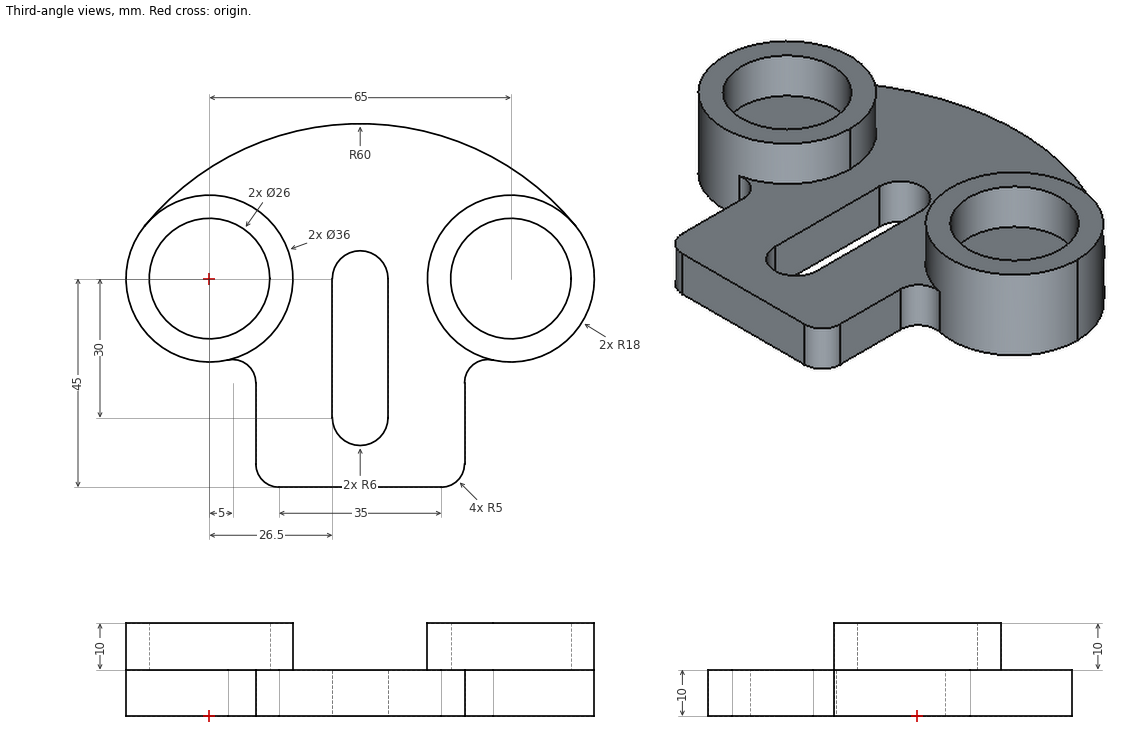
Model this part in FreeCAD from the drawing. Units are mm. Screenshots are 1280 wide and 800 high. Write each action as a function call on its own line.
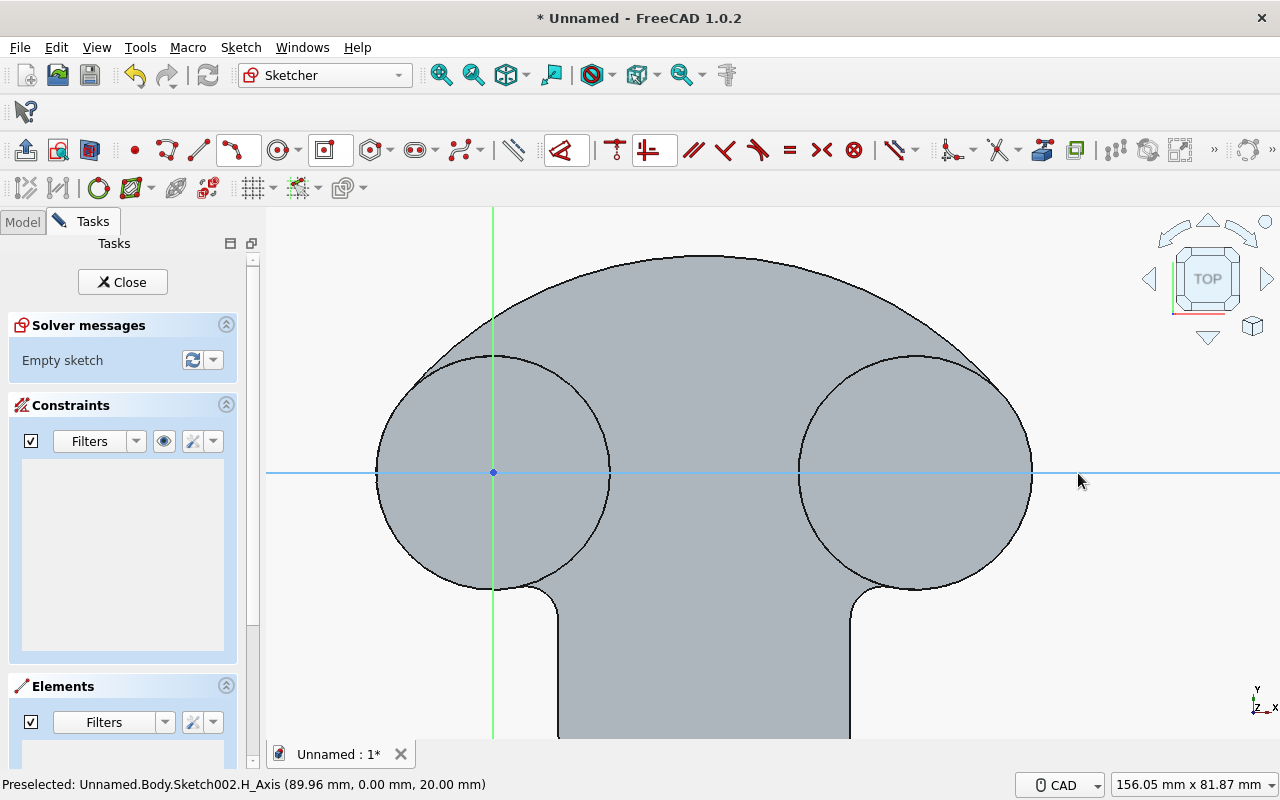
click(278, 150)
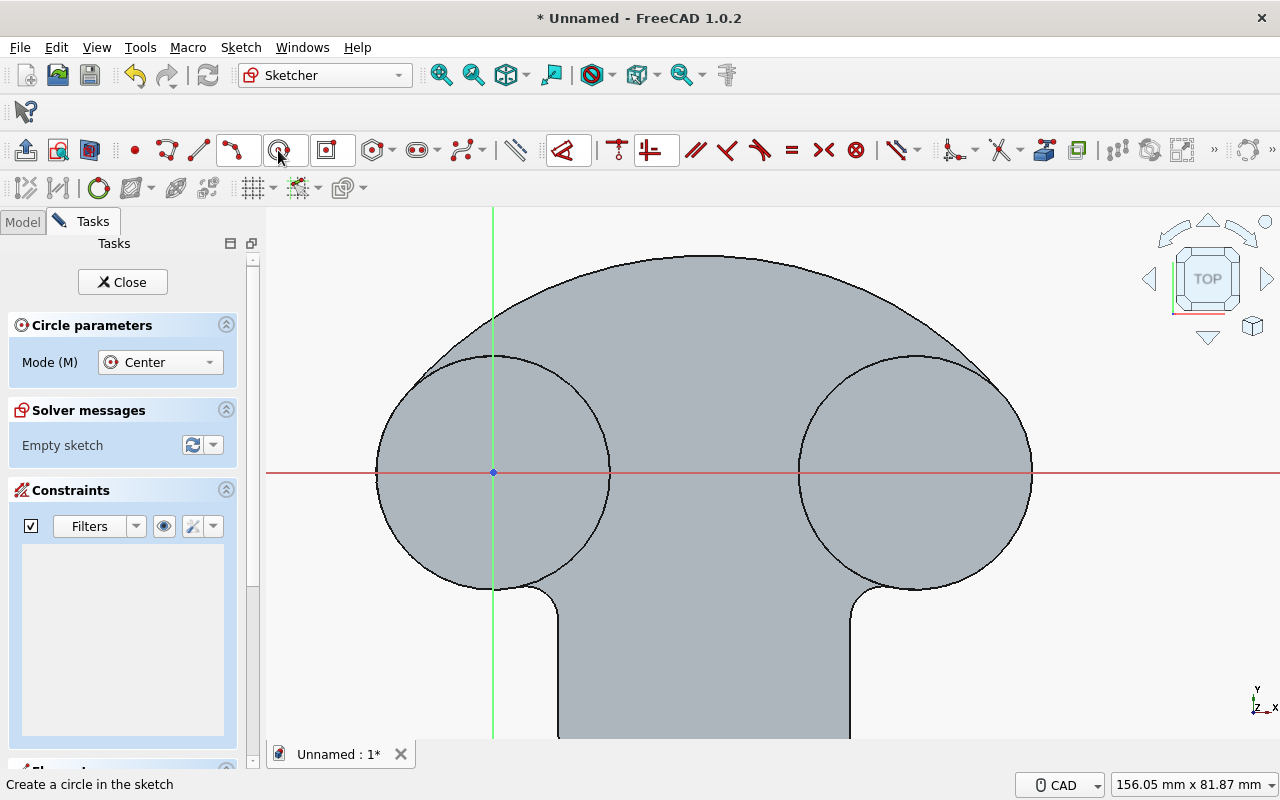
click(493, 473)
move(553, 413)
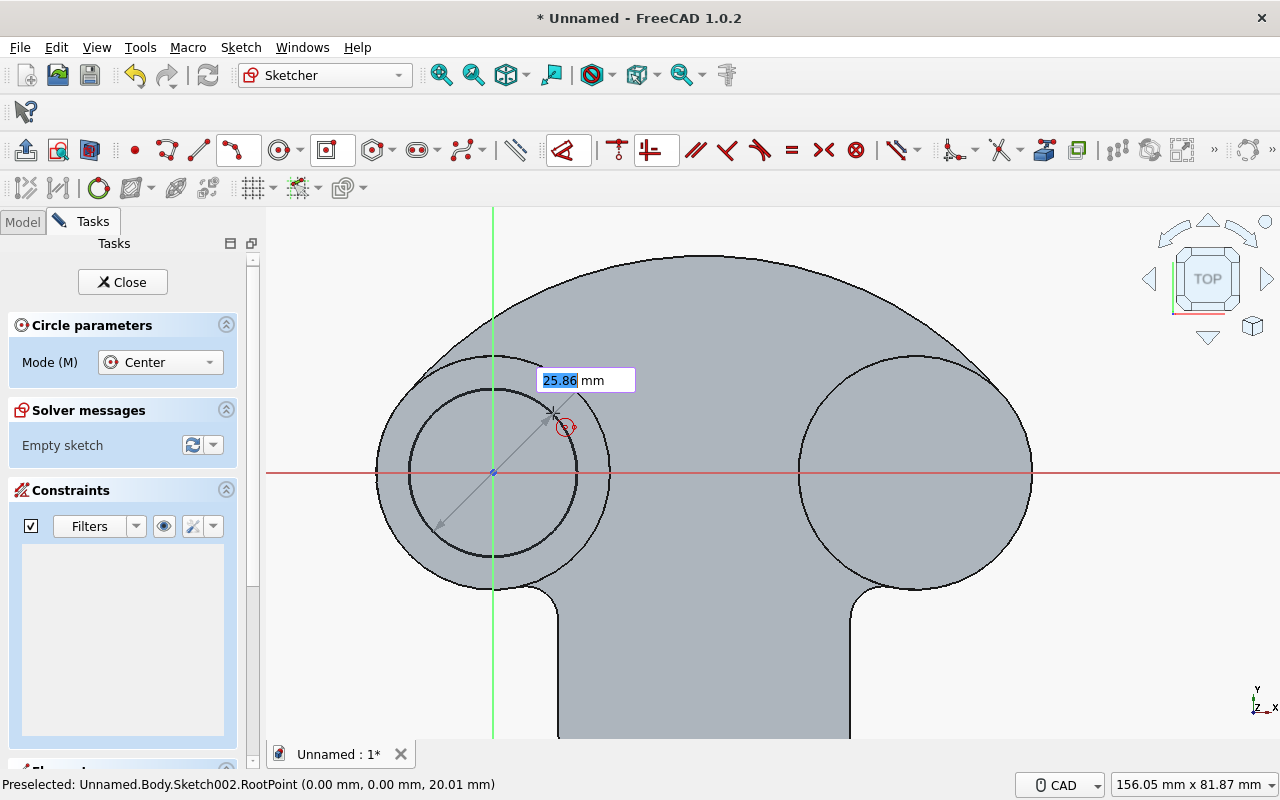
text(26)
key(Return)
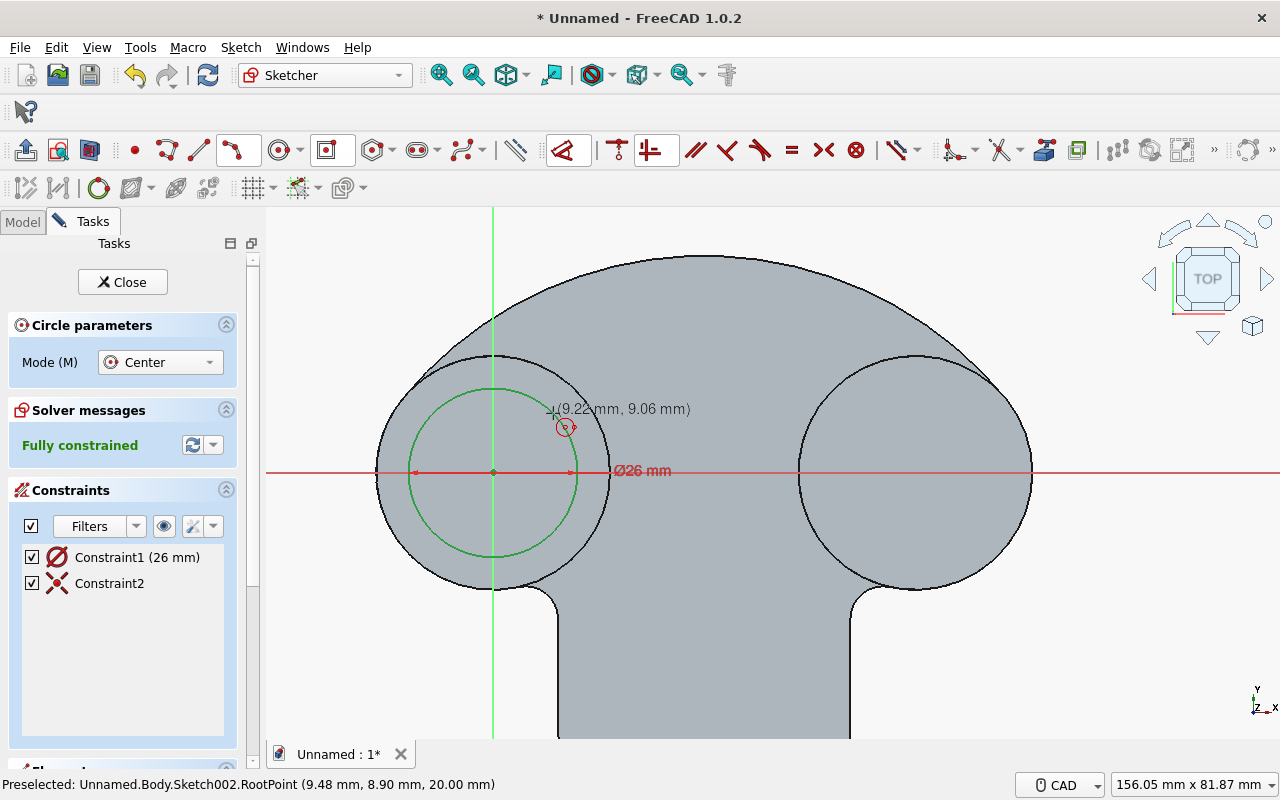
click(915, 473)
move(975, 413)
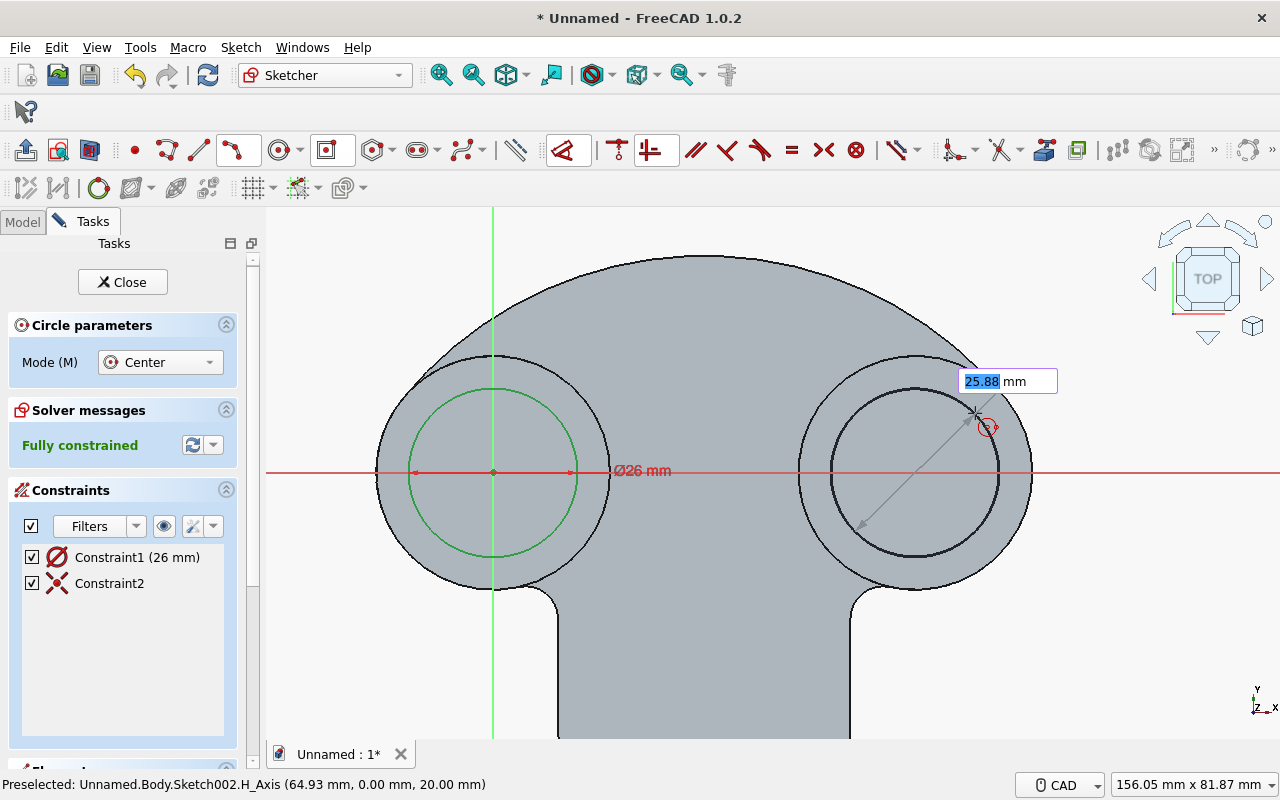
text(26)
key(Return)
key(Escape)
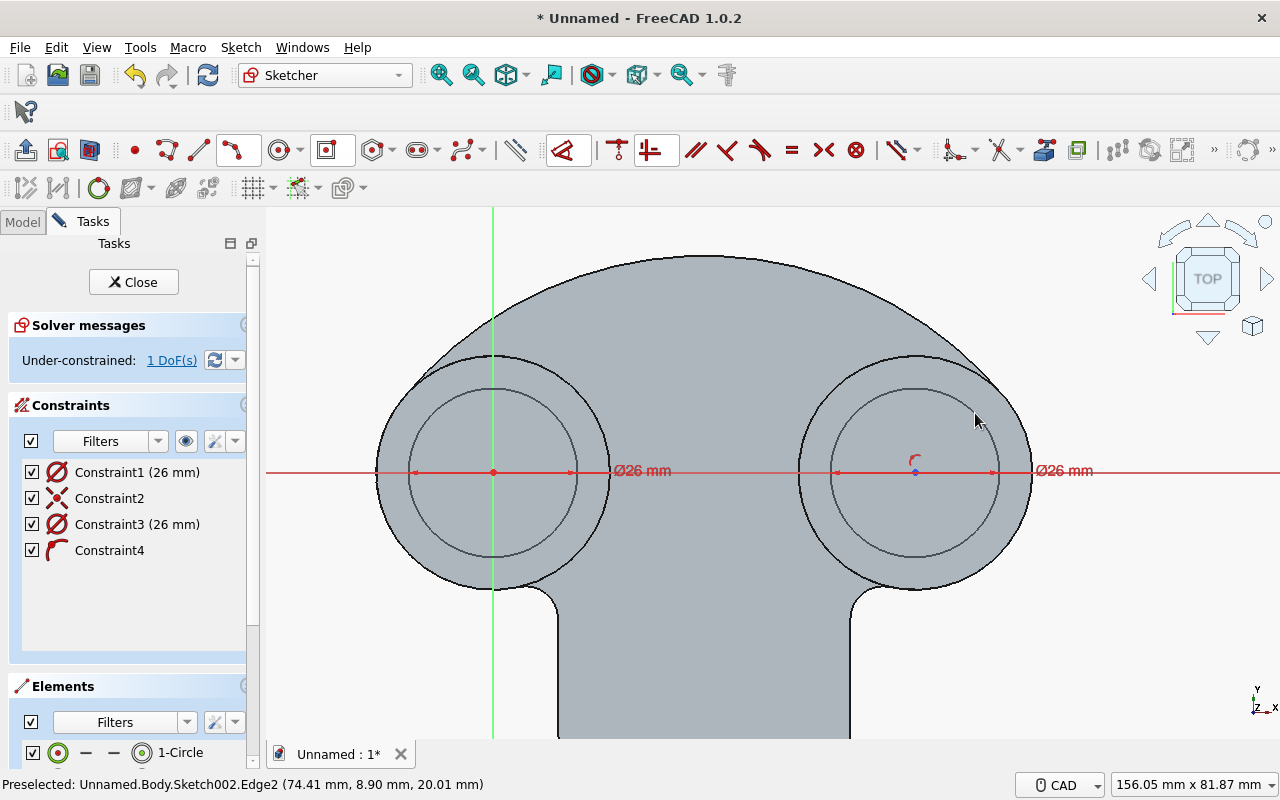
click(915, 473)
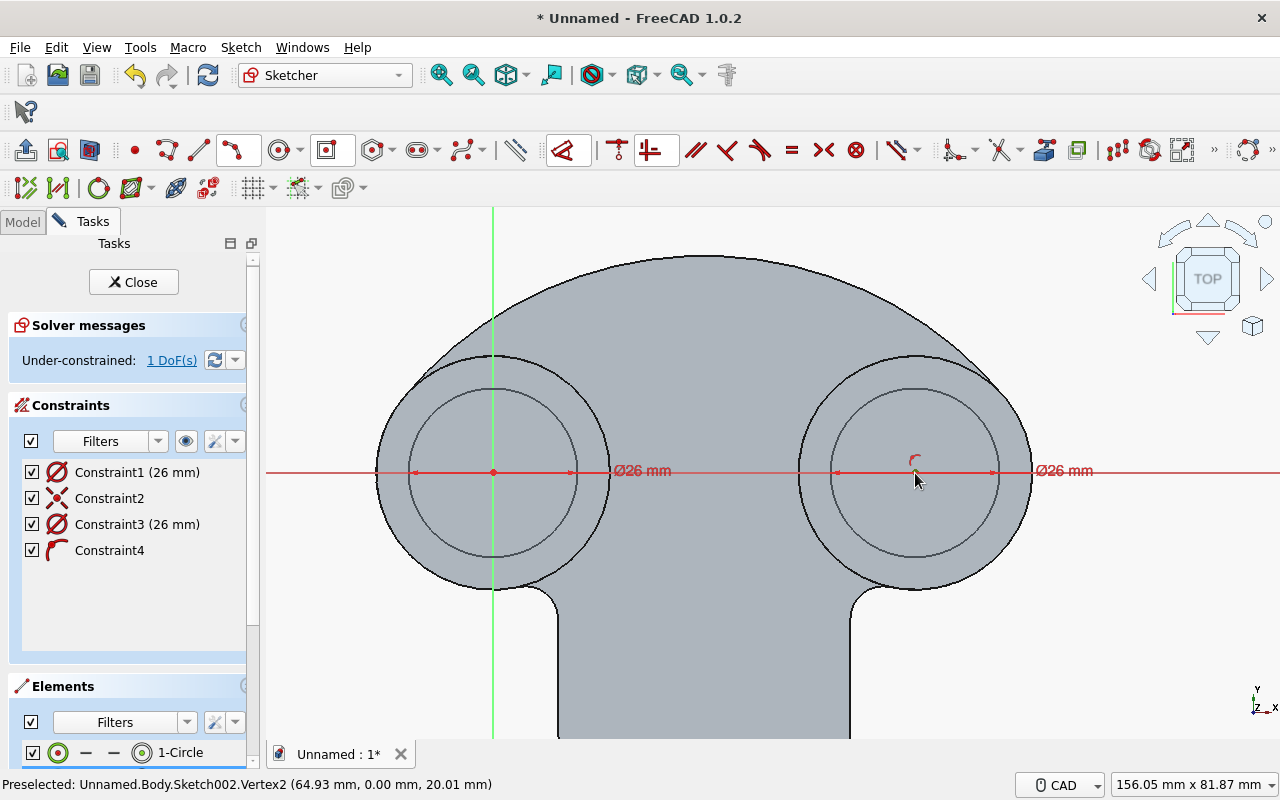
click(586, 150)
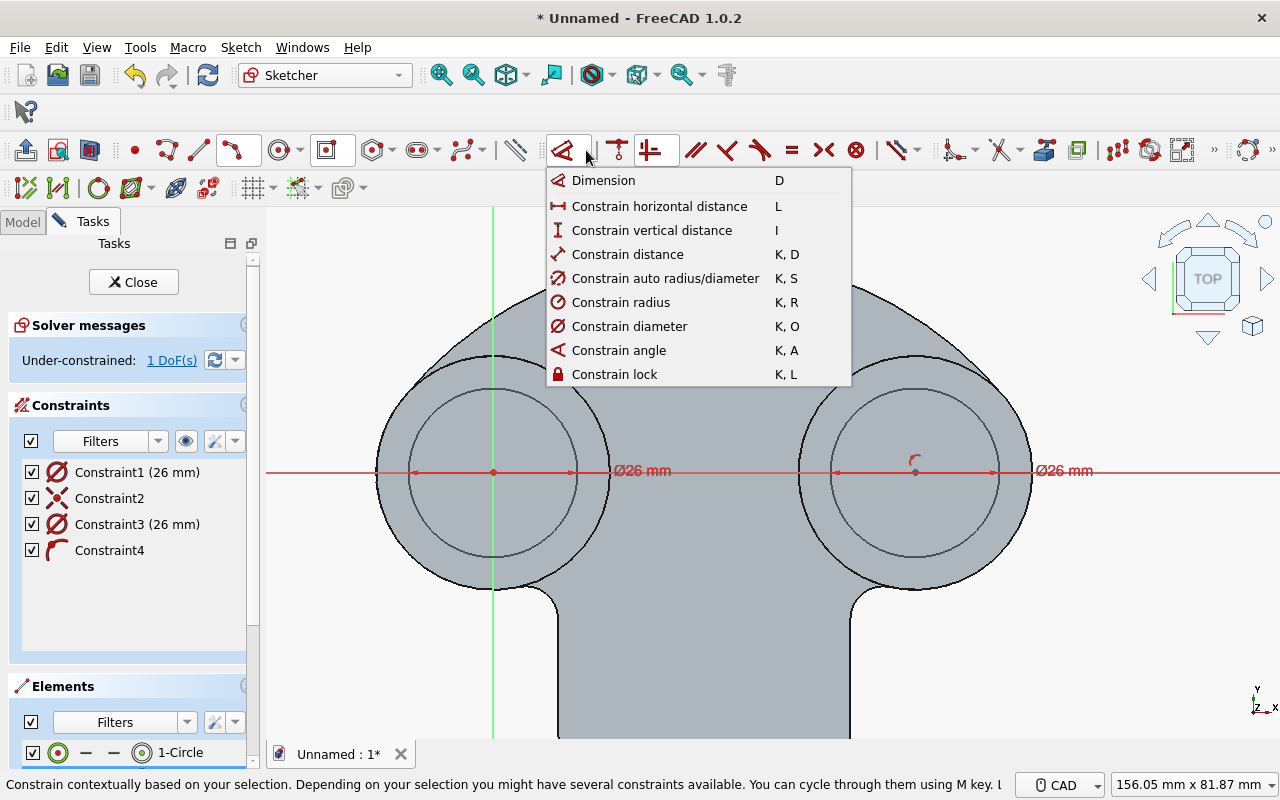
click(699, 206)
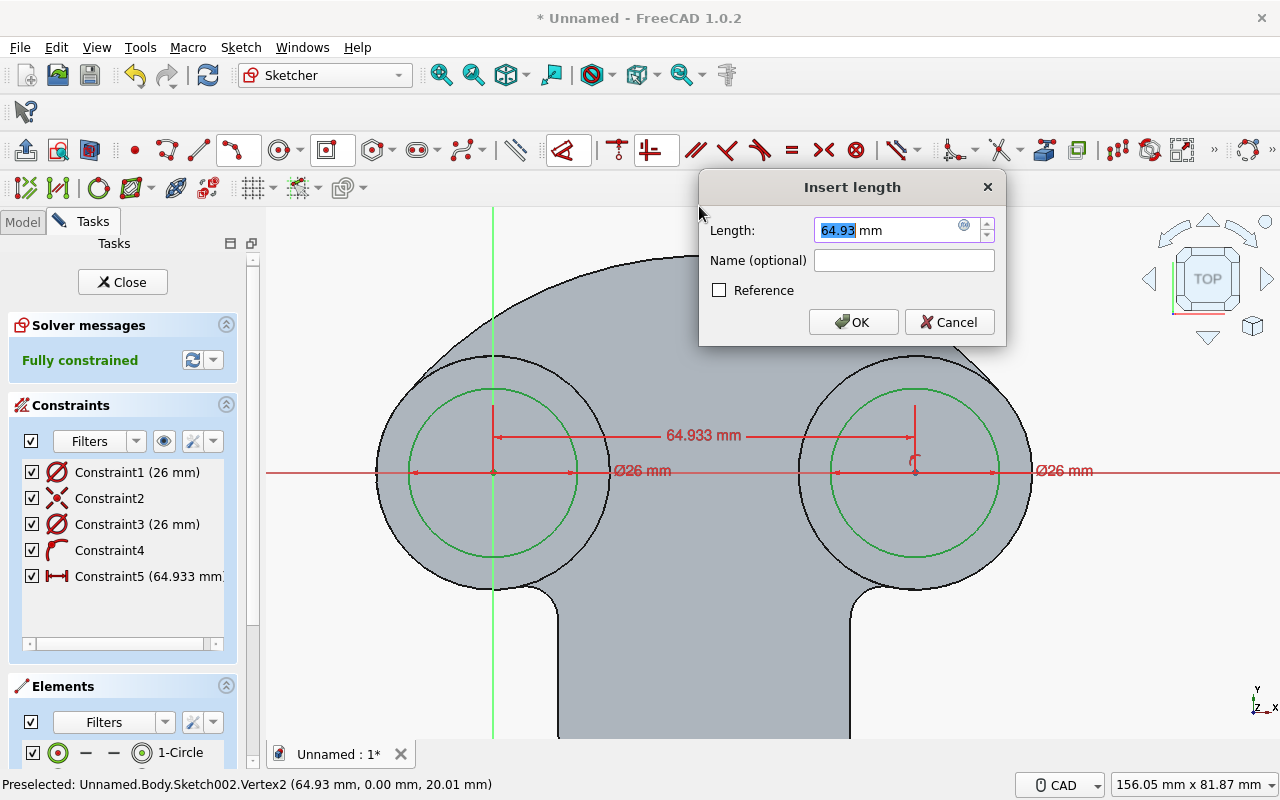
text(65)
key(Return)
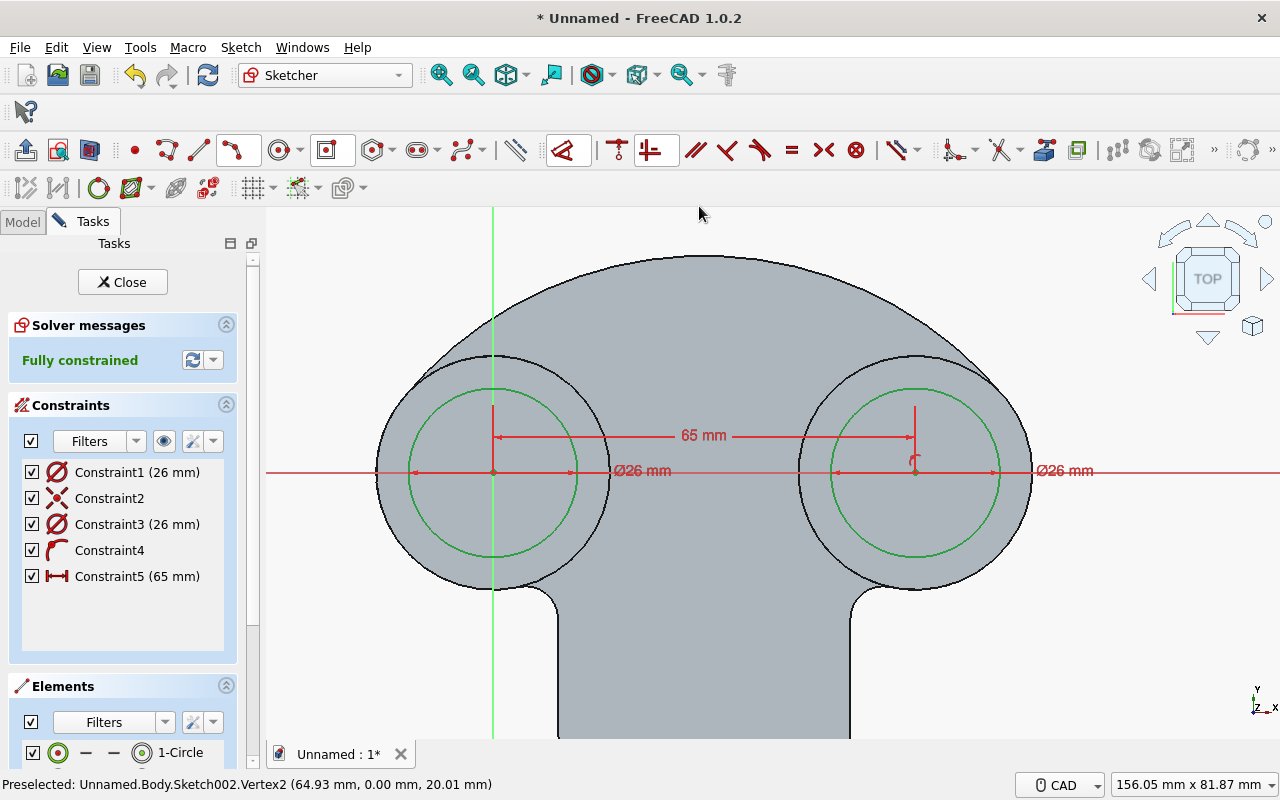
click(123, 282)